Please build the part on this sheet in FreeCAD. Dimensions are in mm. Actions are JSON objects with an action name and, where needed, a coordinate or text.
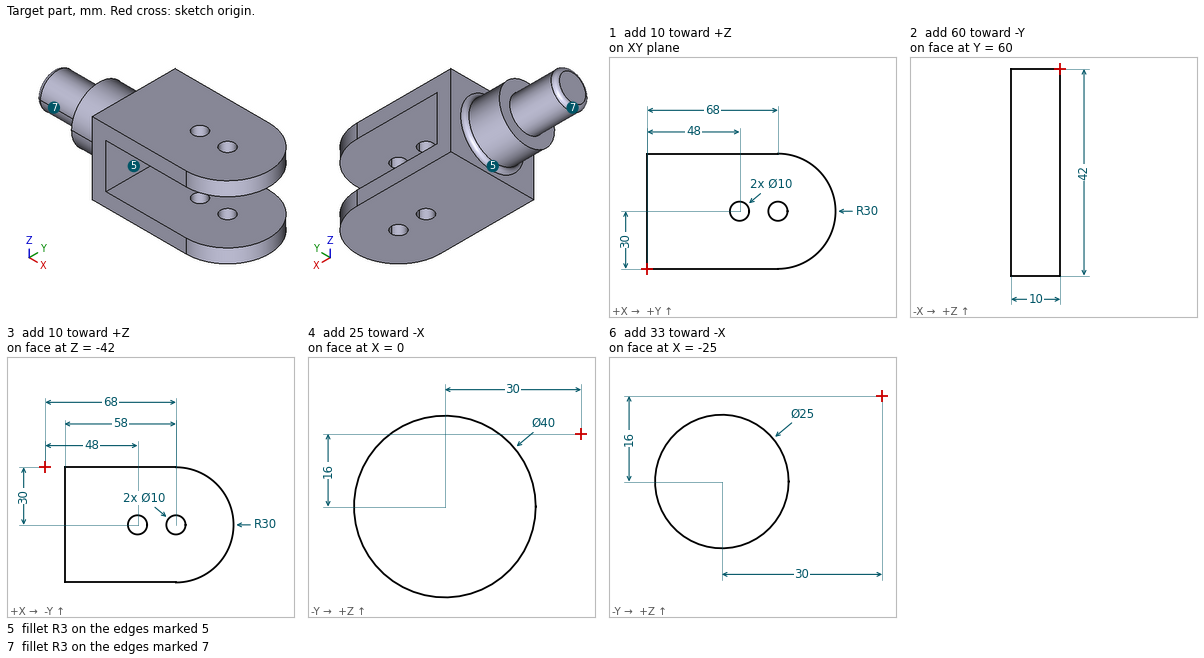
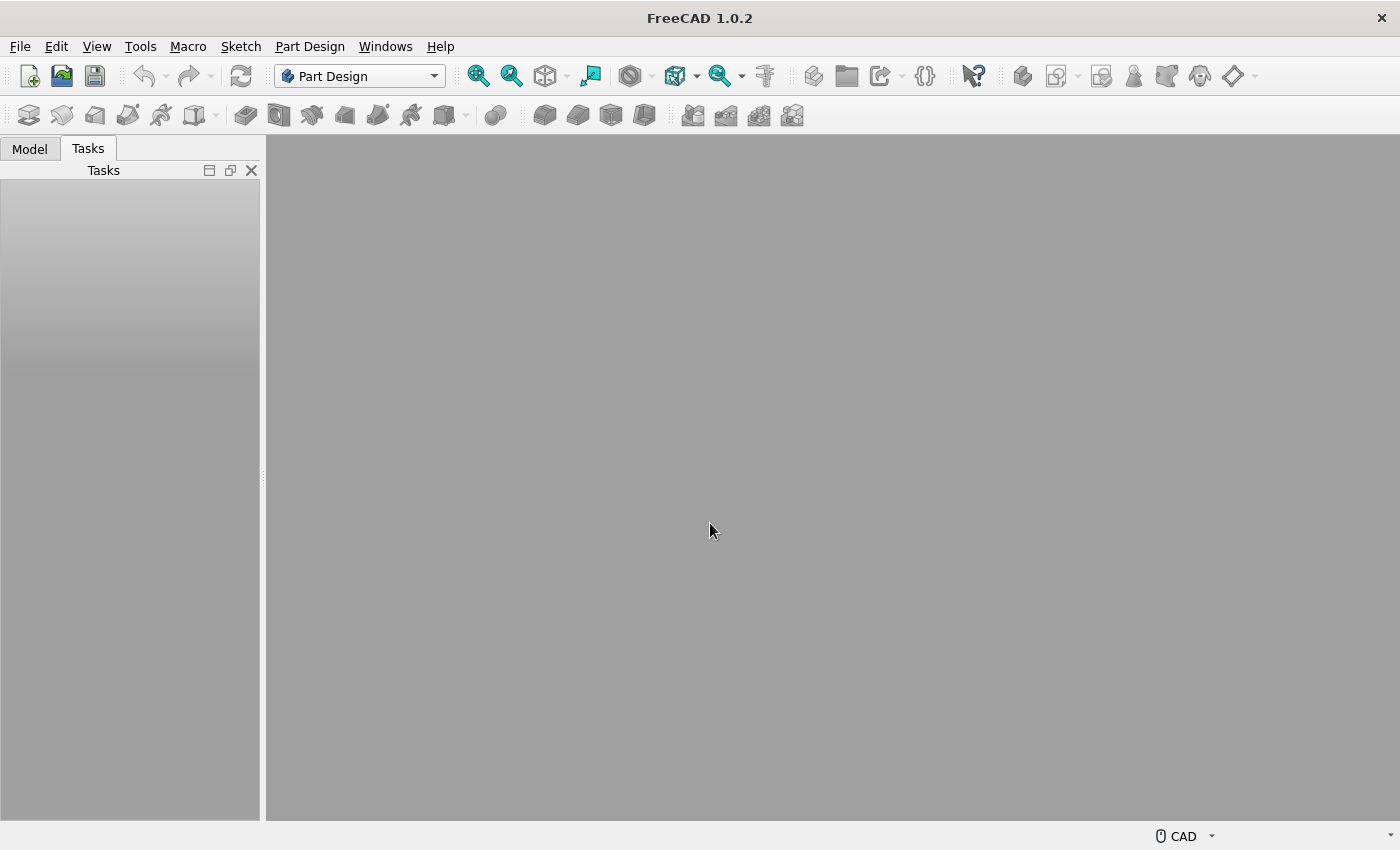
{"action": "left_click", "coordinate": [29, 76]}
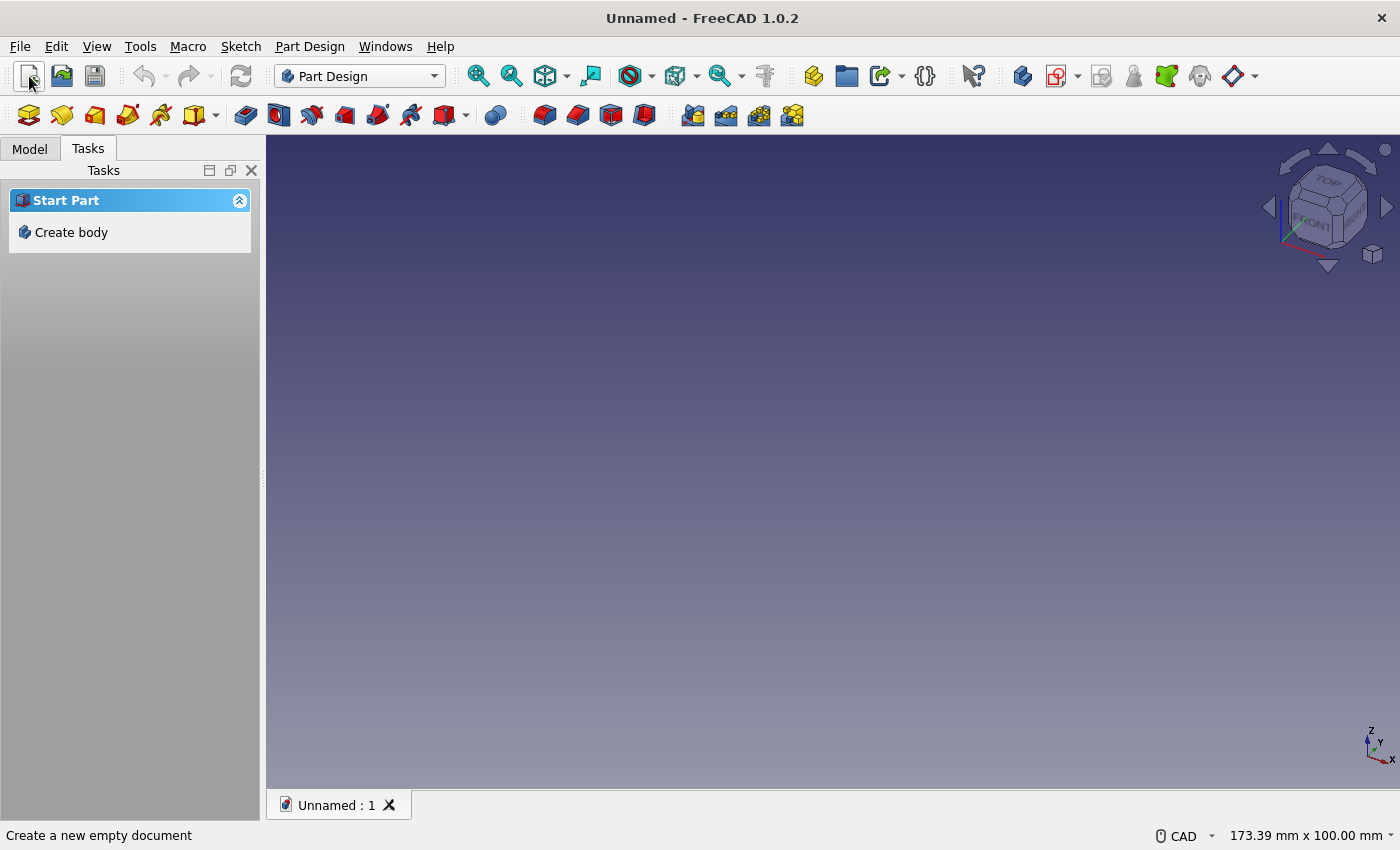
{"action": "left_click", "coordinate": [1056, 76]}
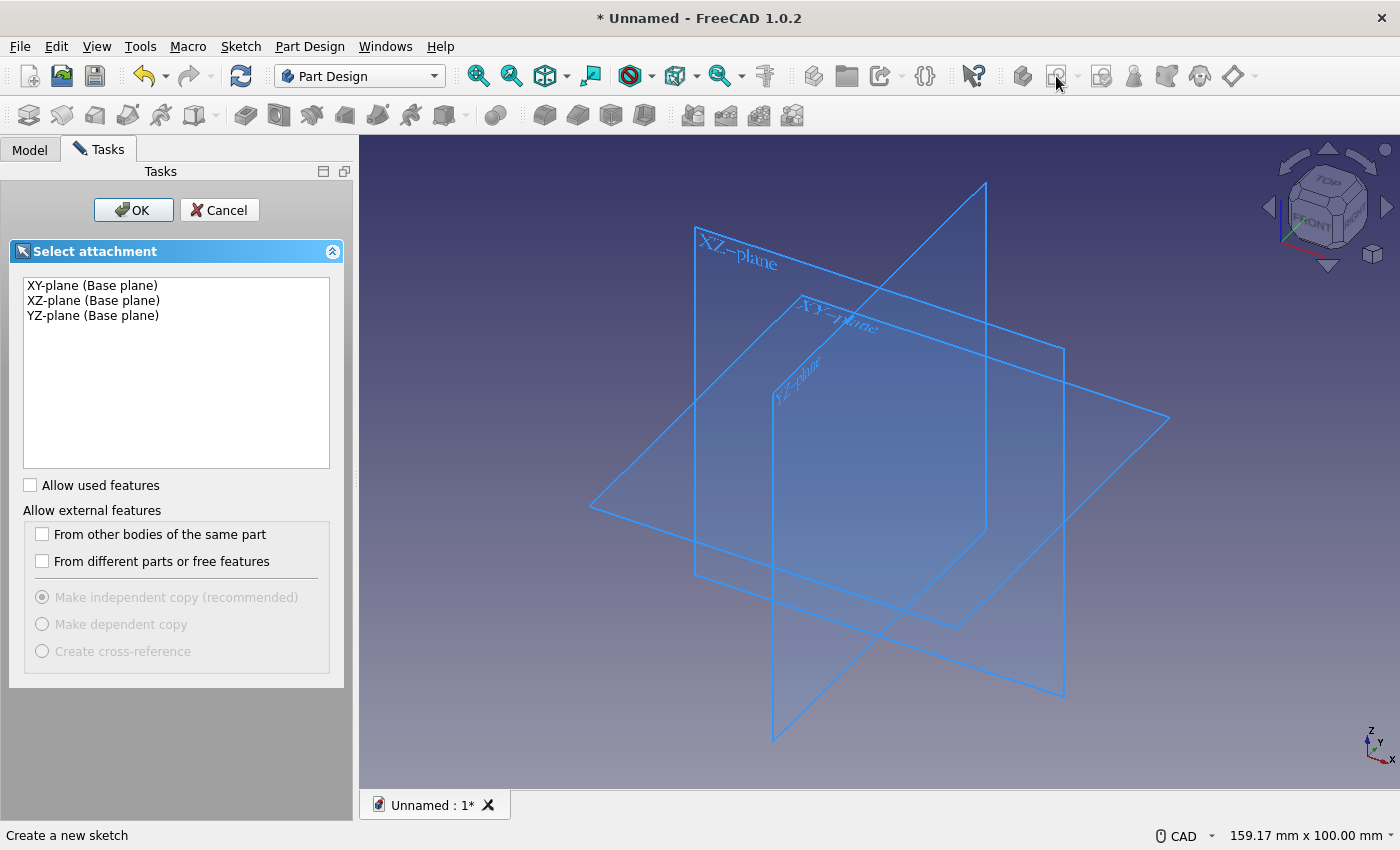
{"action": "left_click", "coordinate": [84, 286]}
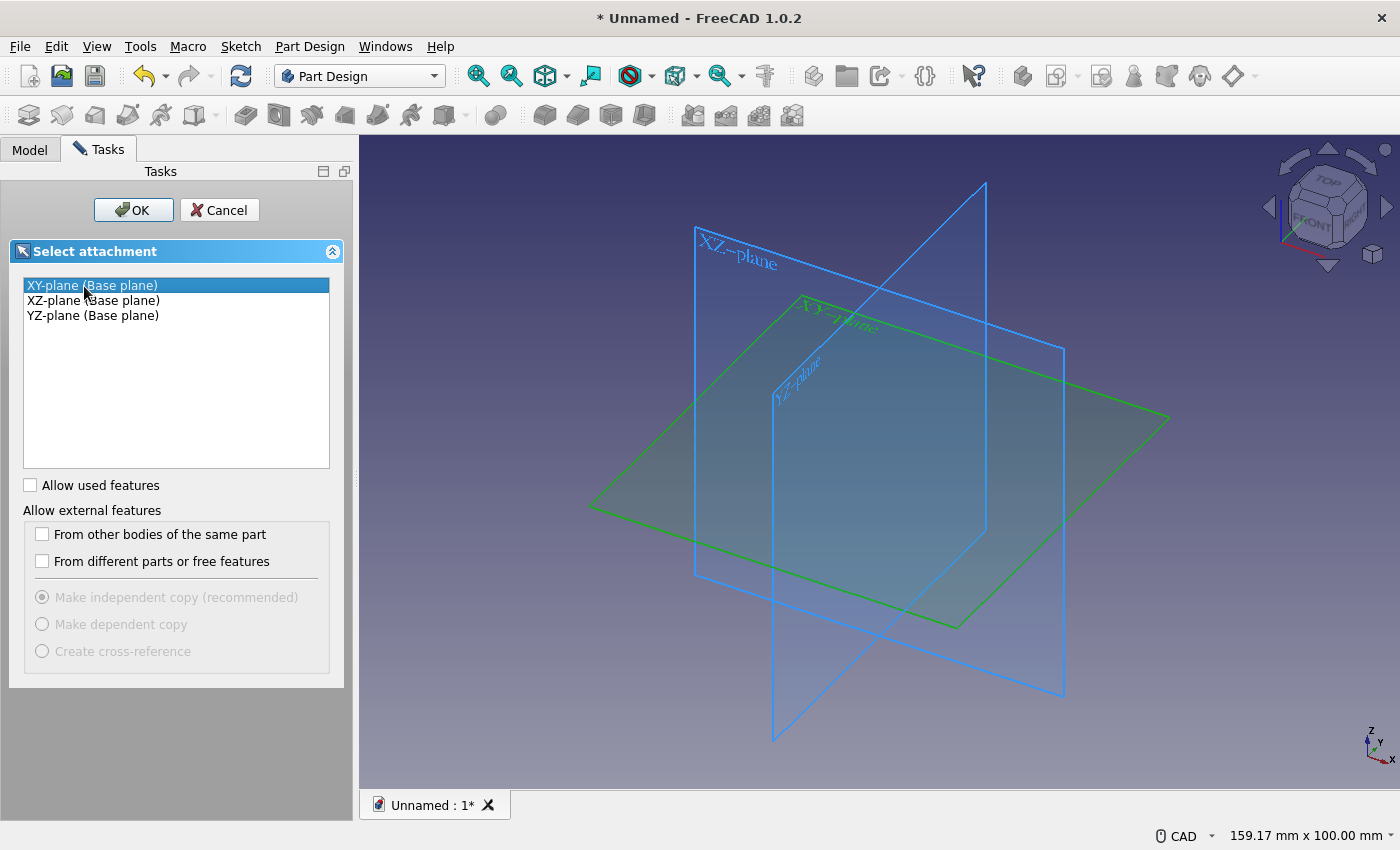
{"action": "left_click", "coordinate": [134, 210]}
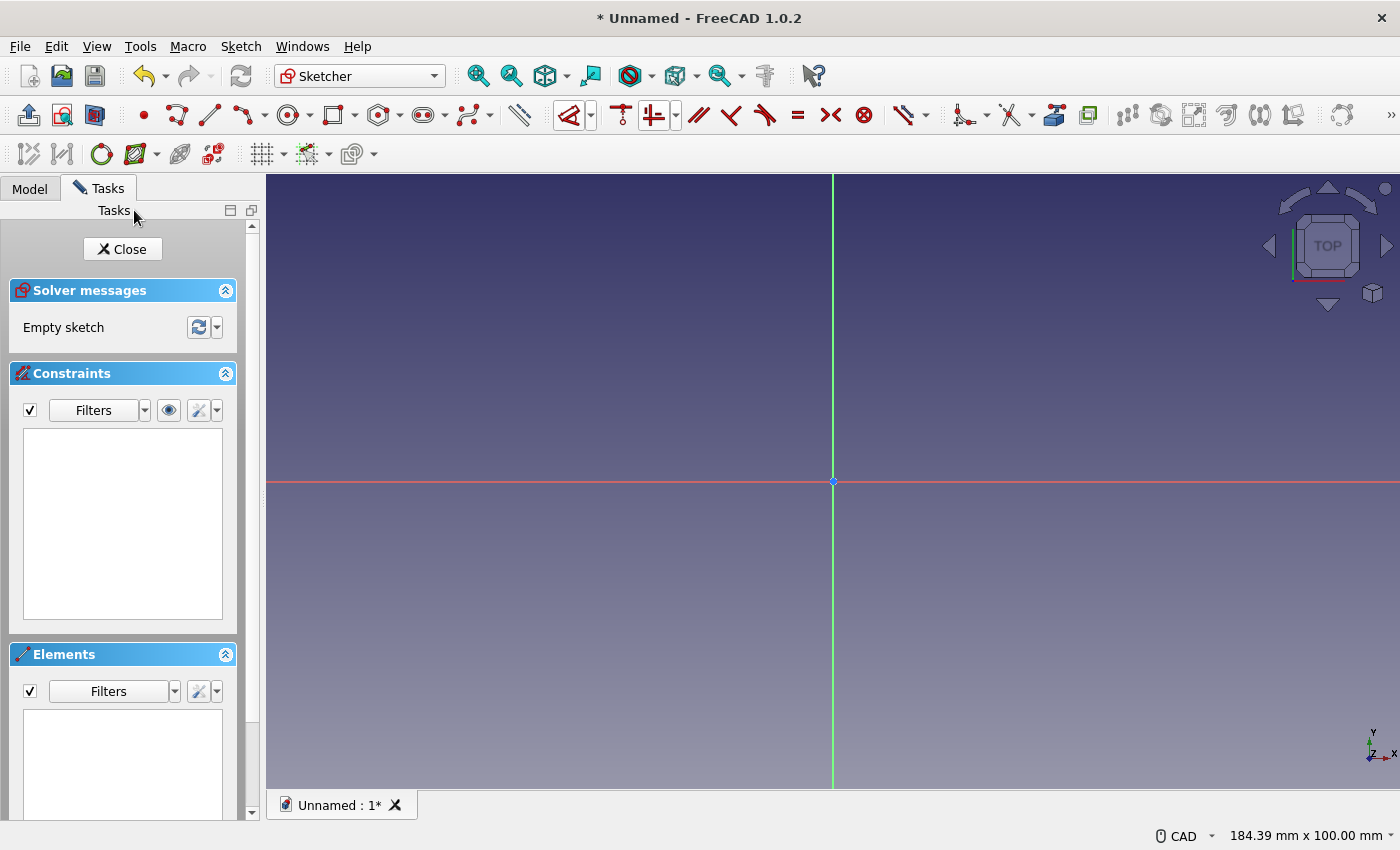
{"action": "scroll", "coordinate": [294, 761], "scroll_direction": "down", "scroll_amount": 2}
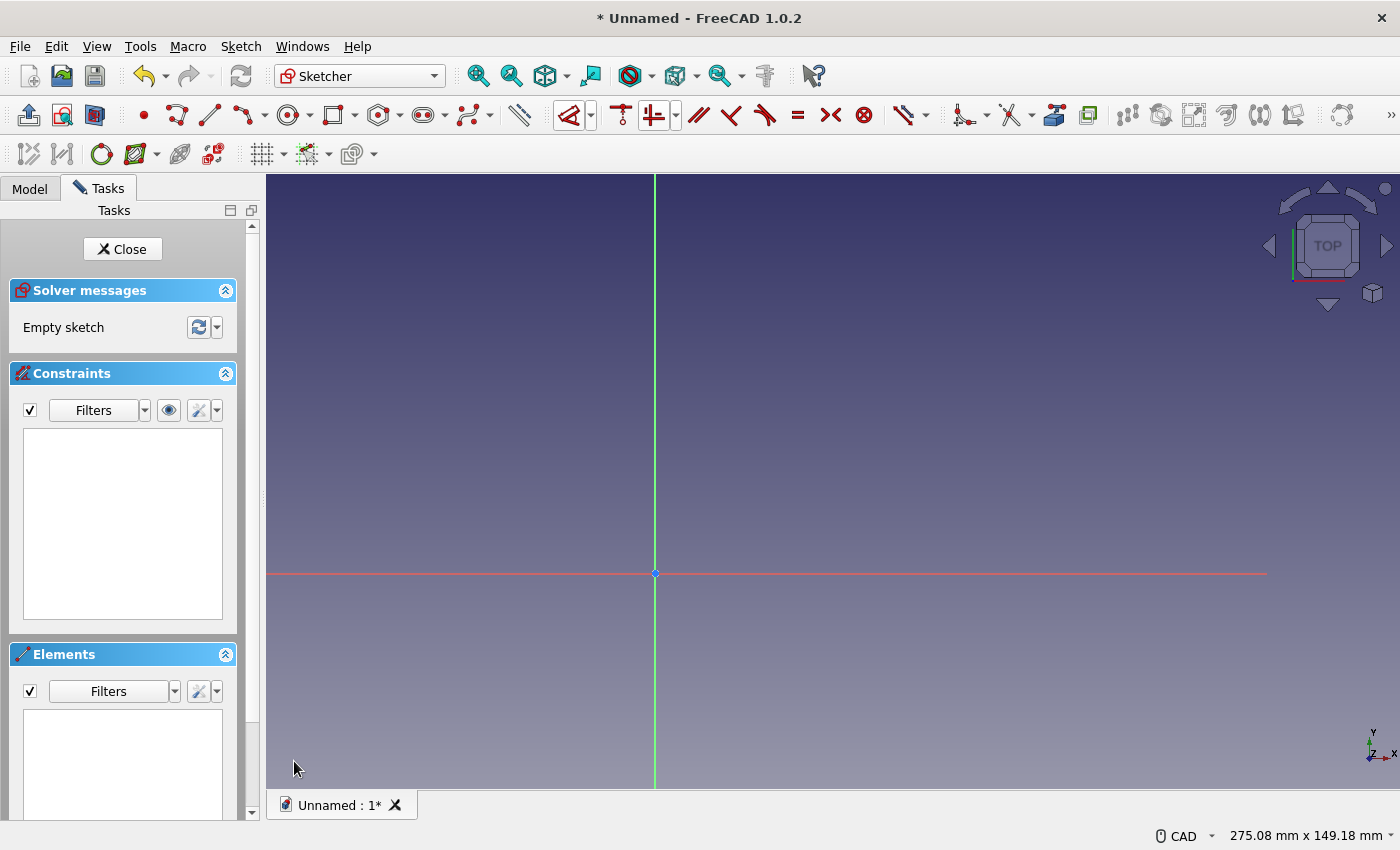
{"action": "scroll", "coordinate": [1046, 387], "scroll_direction": "up", "scroll_amount": 2}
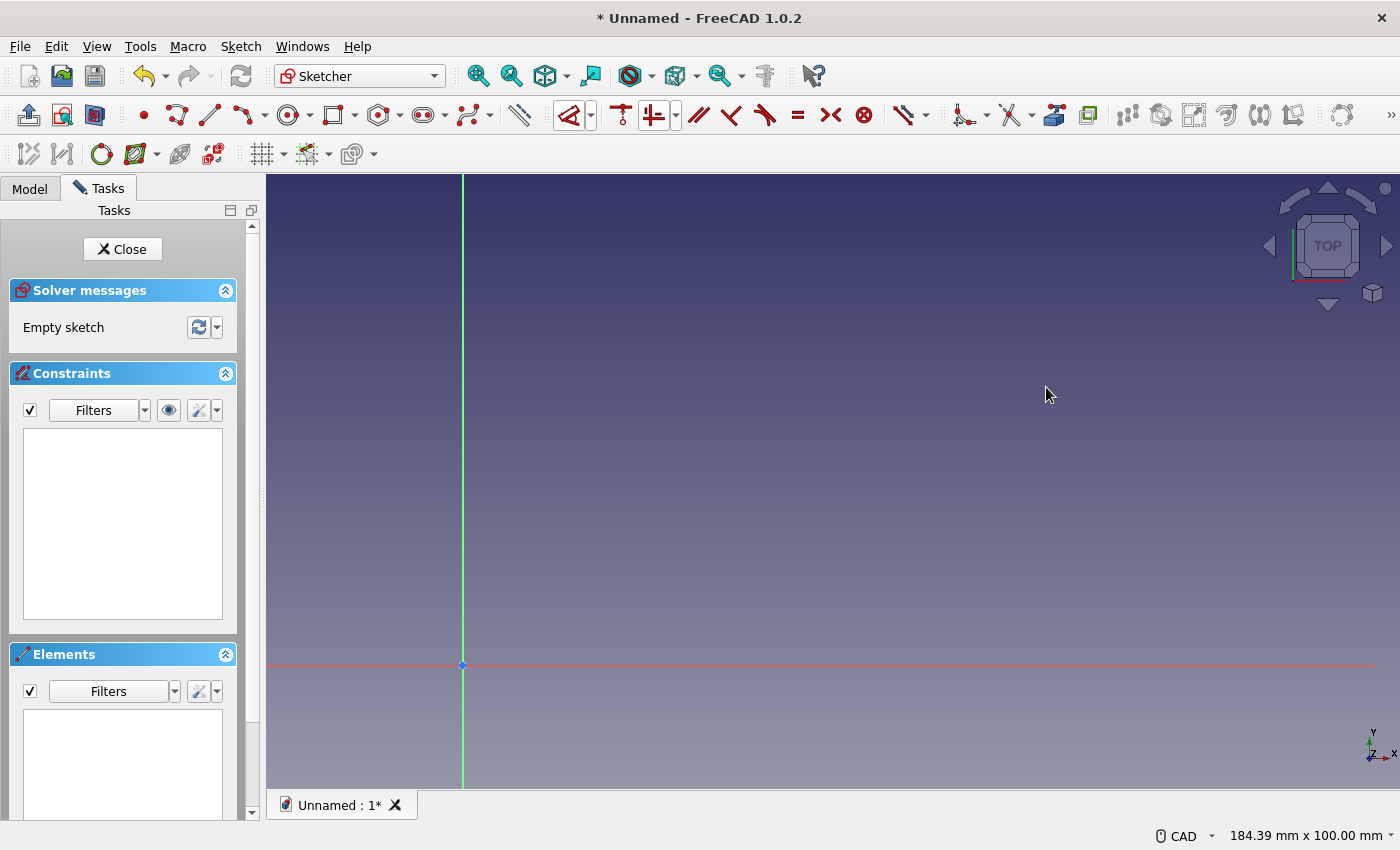
{"action": "key", "text": "g m"}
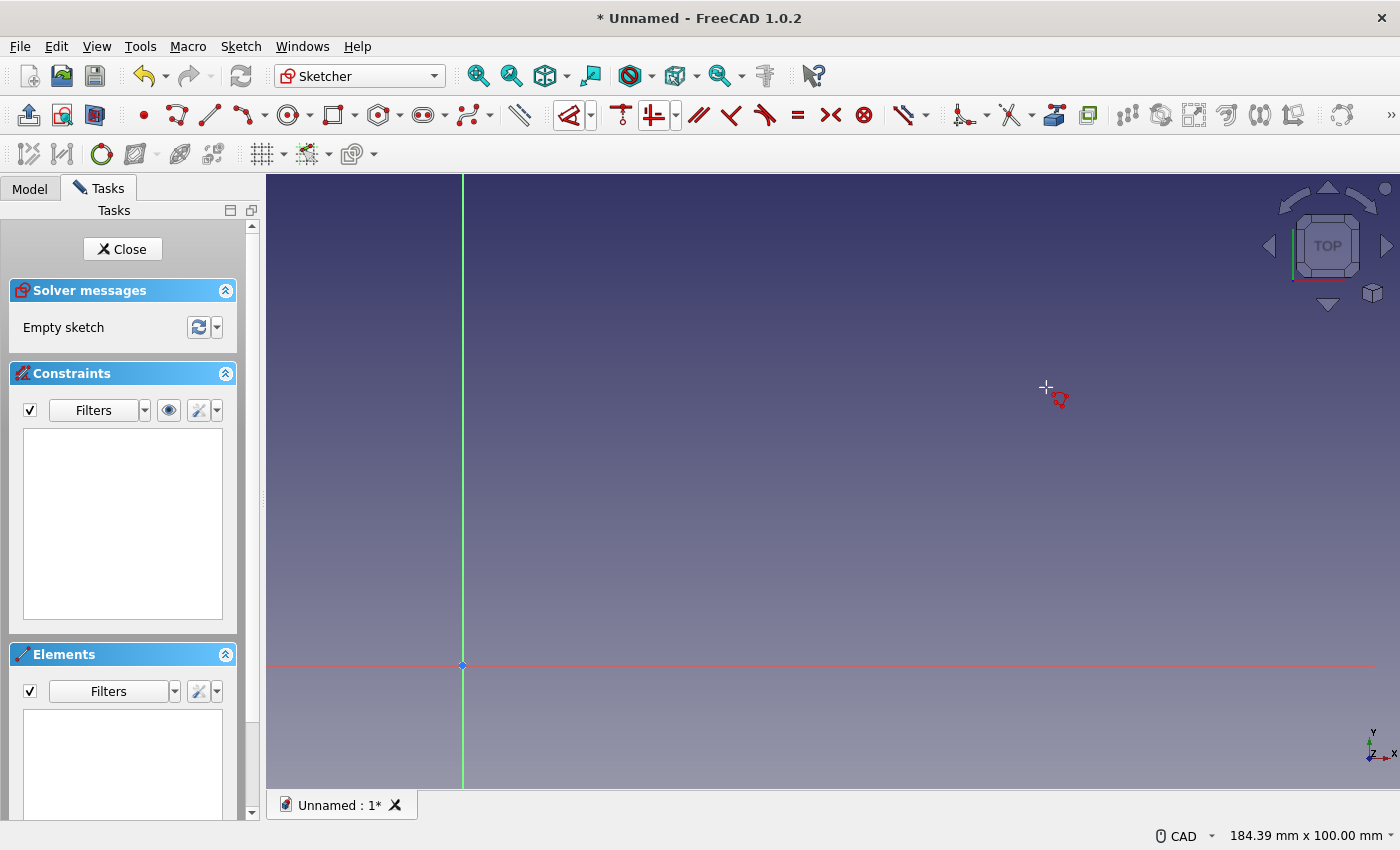
{"action": "left_click", "coordinate": [881, 297]}
{"action": "left_click", "coordinate": [463, 297]}
{"action": "left_click", "coordinate": [463, 666]}
{"action": "left_click", "coordinate": [881, 657]}
{"action": "right_click", "coordinate": [881, 657]}